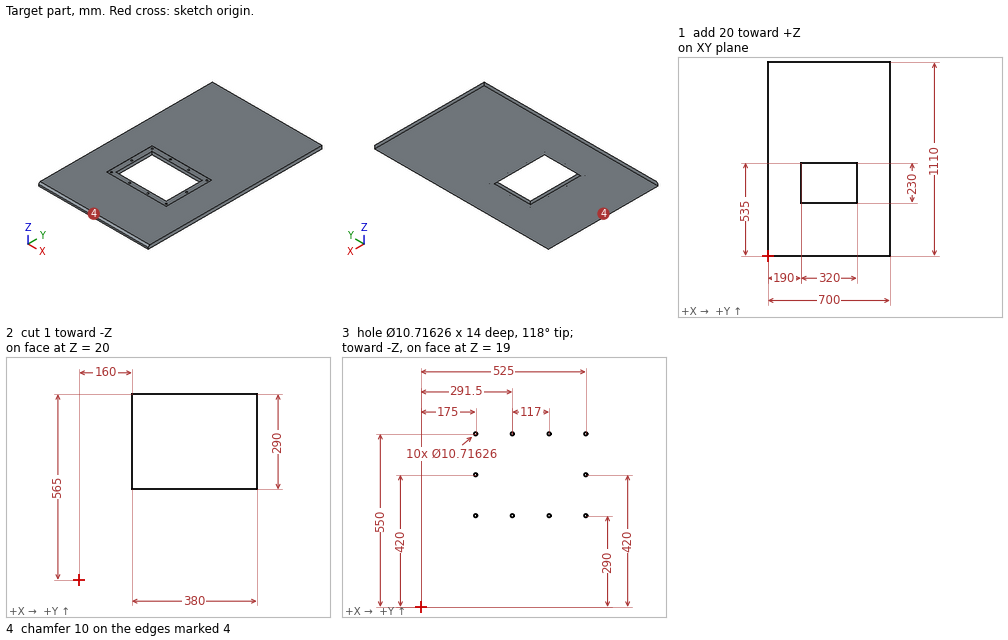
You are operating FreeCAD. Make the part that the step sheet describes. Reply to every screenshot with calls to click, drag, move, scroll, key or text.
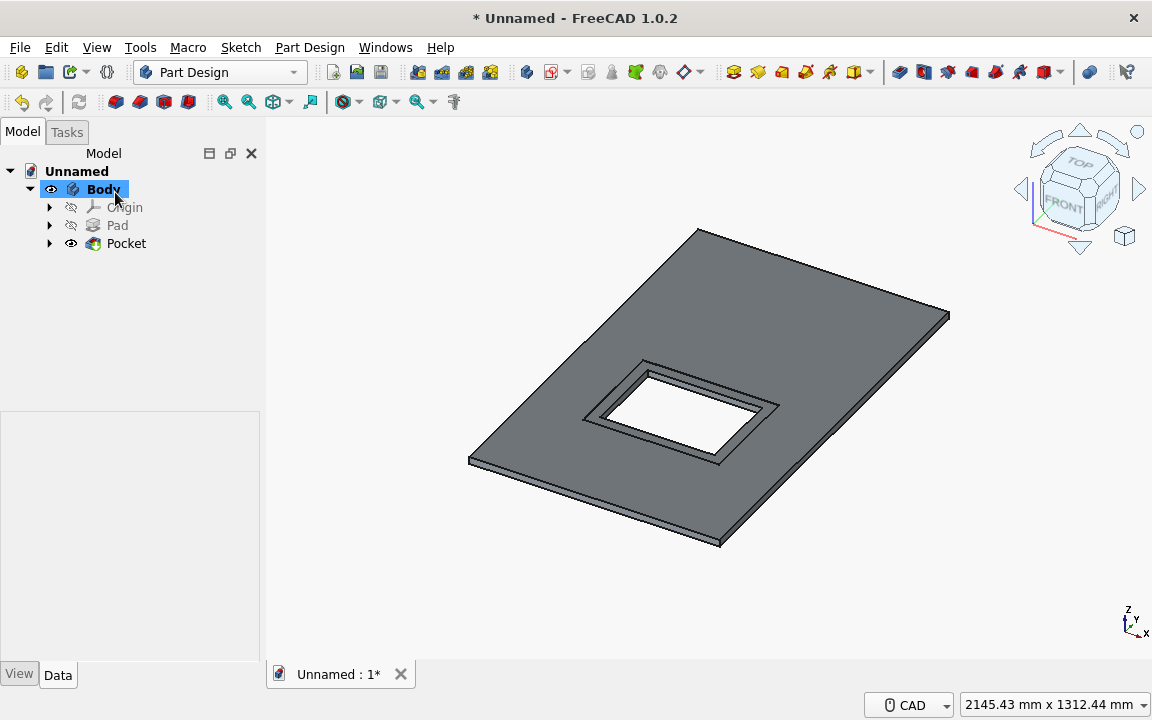
scroll(714, 456, up, 6)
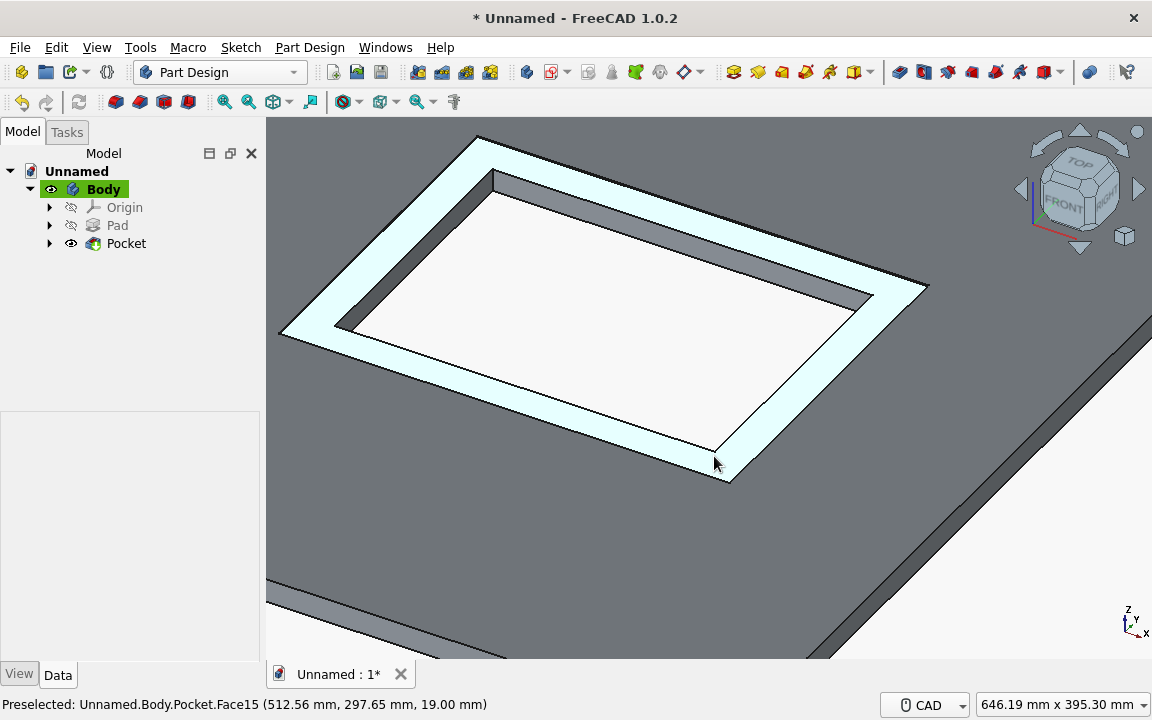
click(712, 458)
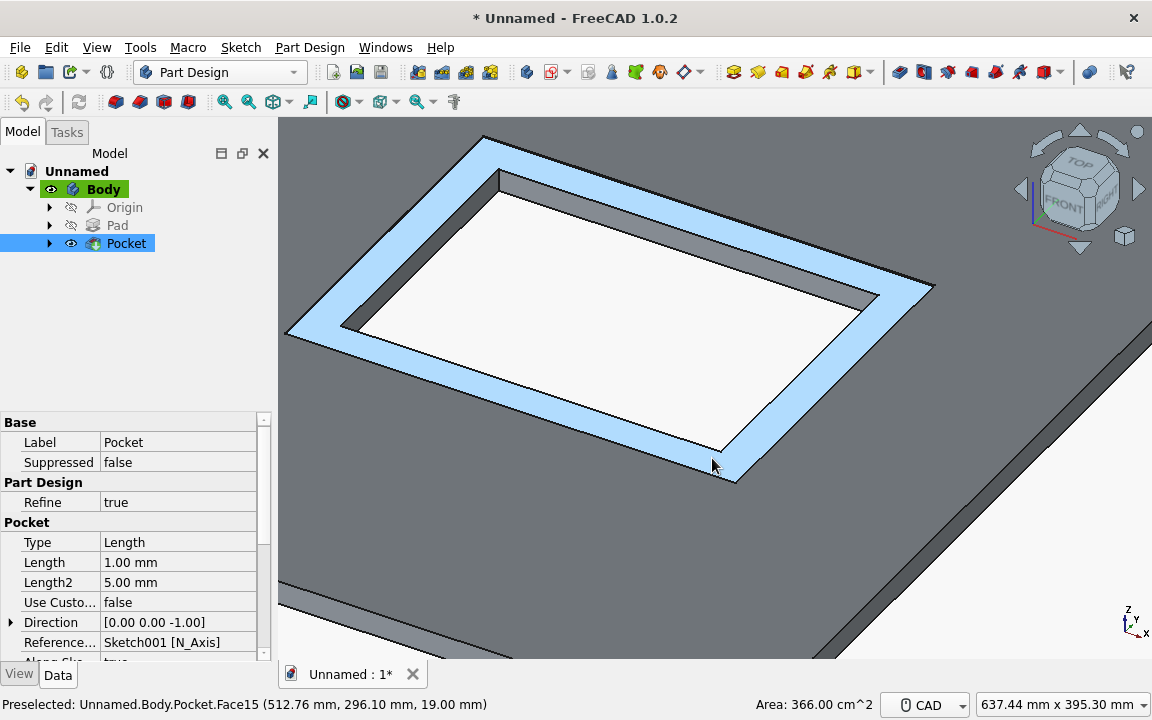
click(552, 72)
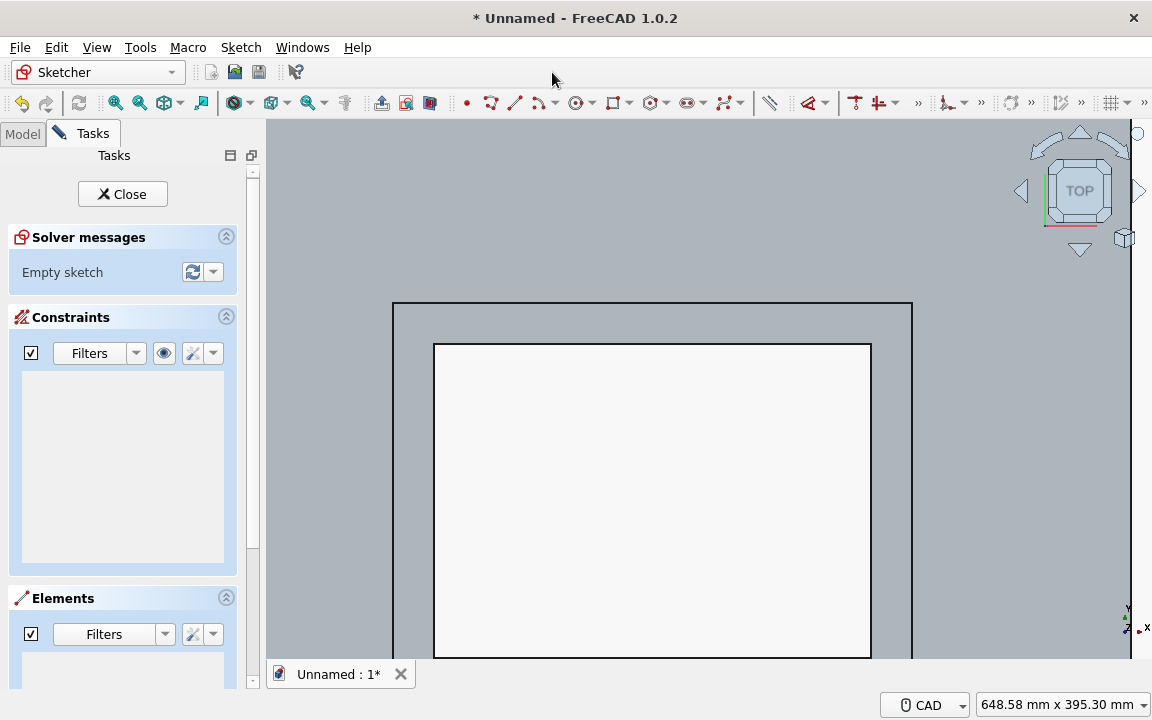
scroll(725, 147, down, 4)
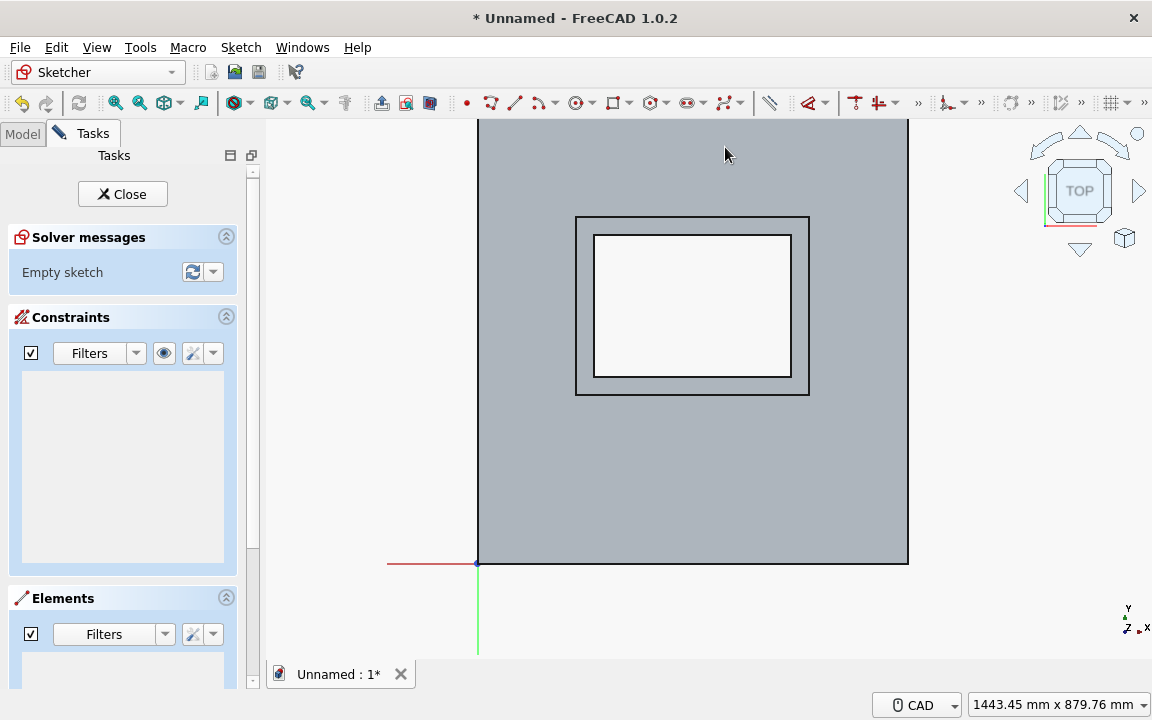
click(576, 104)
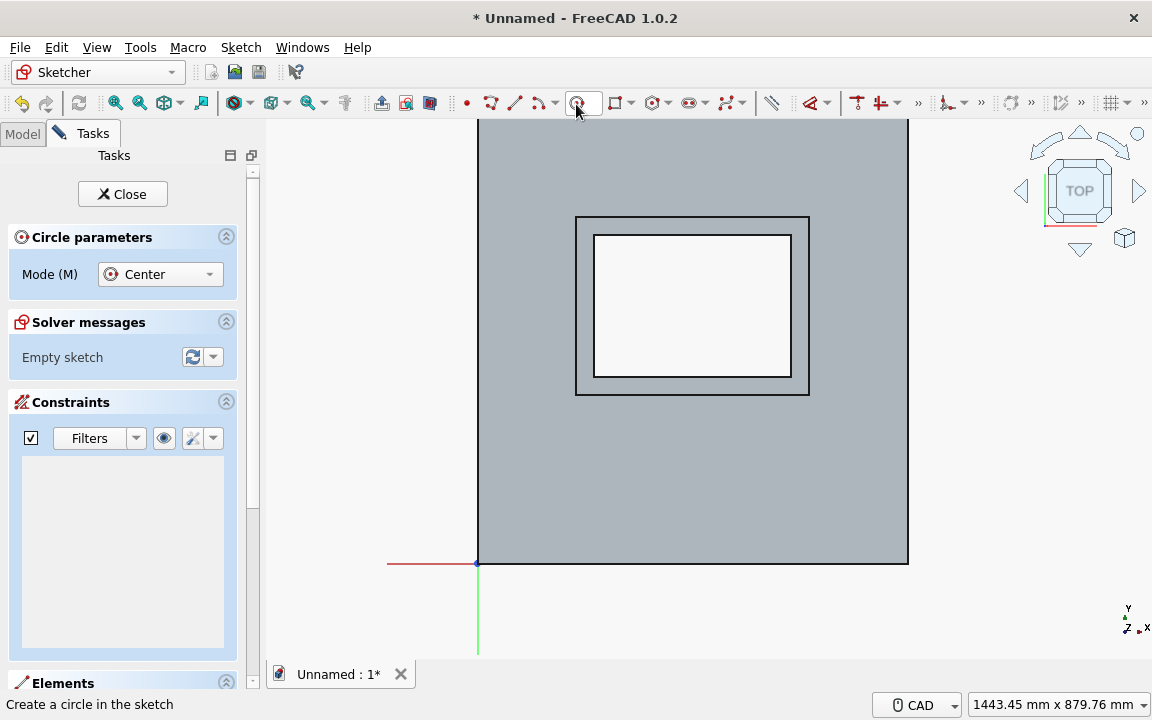
scroll(585, 226, up, 10)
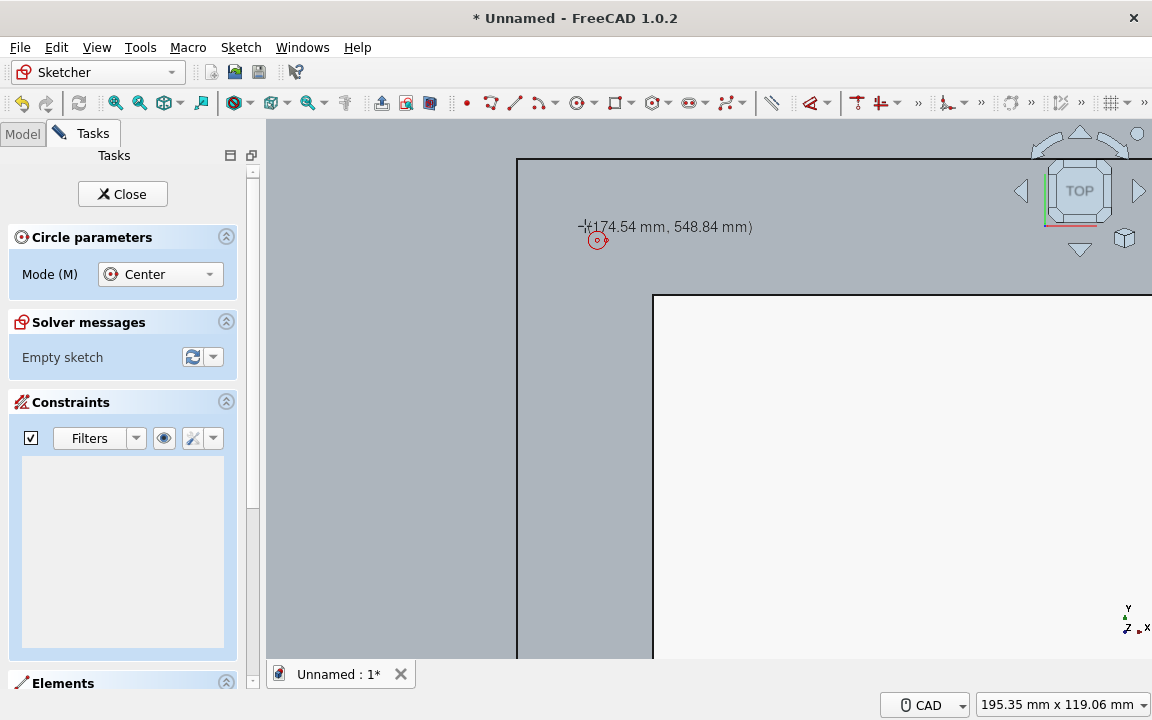
scroll(585, 221, down, 10)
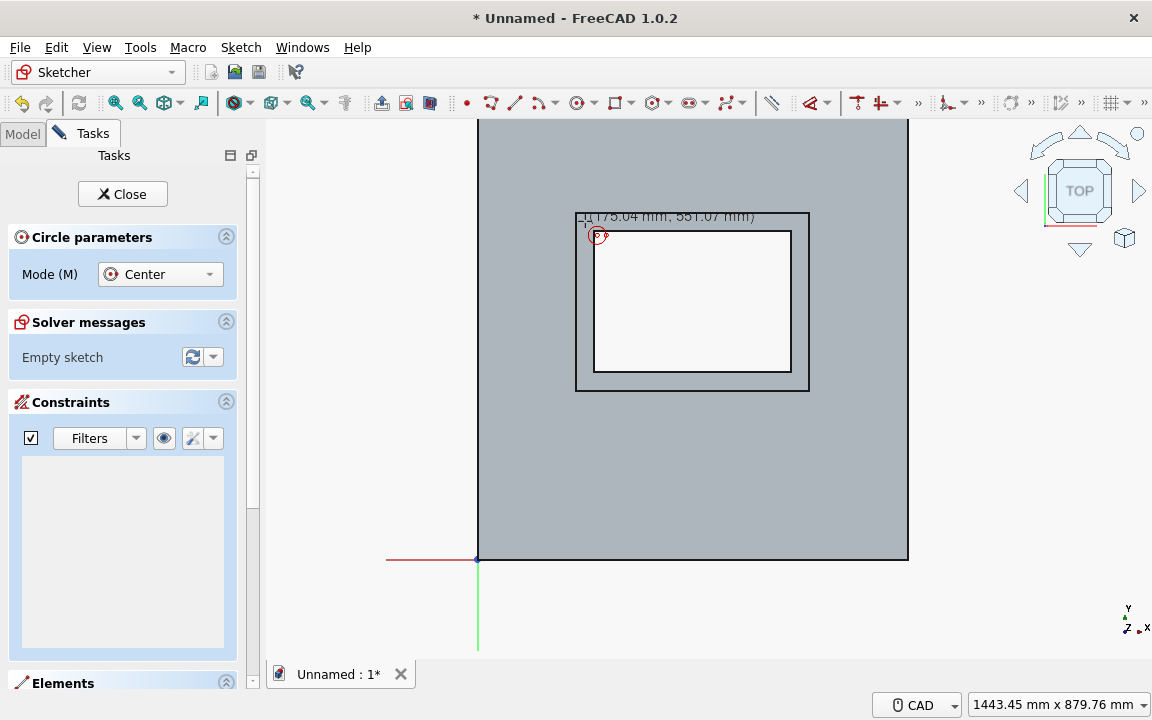
click(585, 222)
move(588, 220)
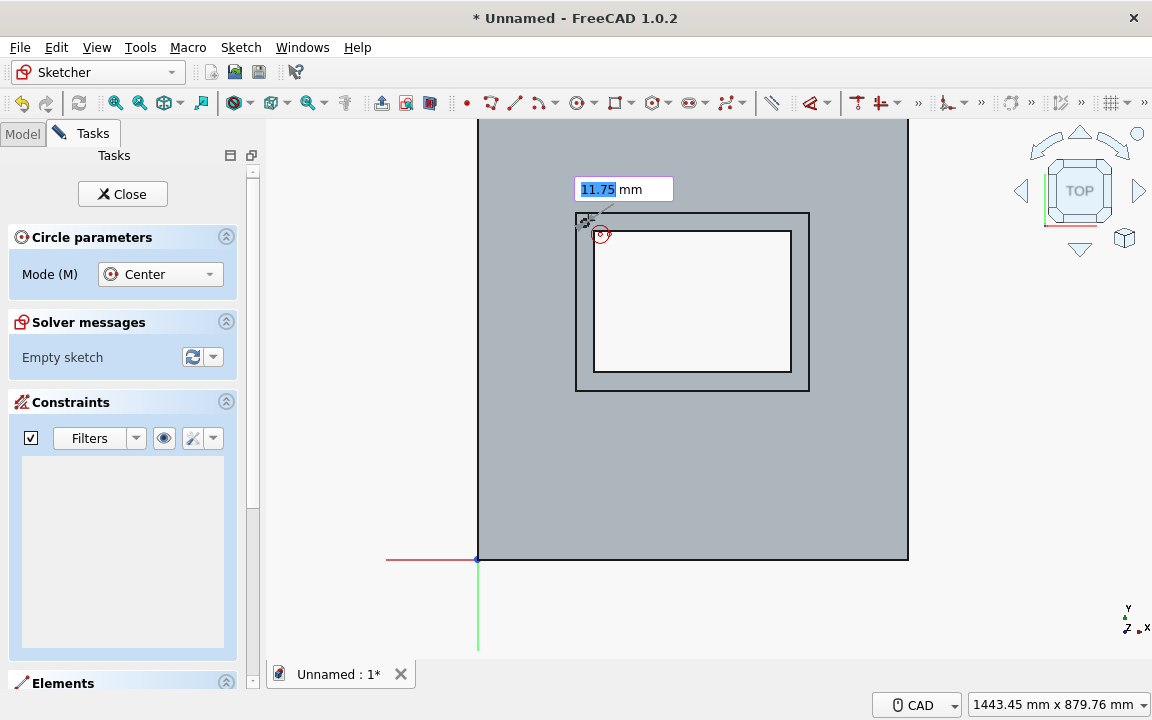
text(10.71626)
key(Return)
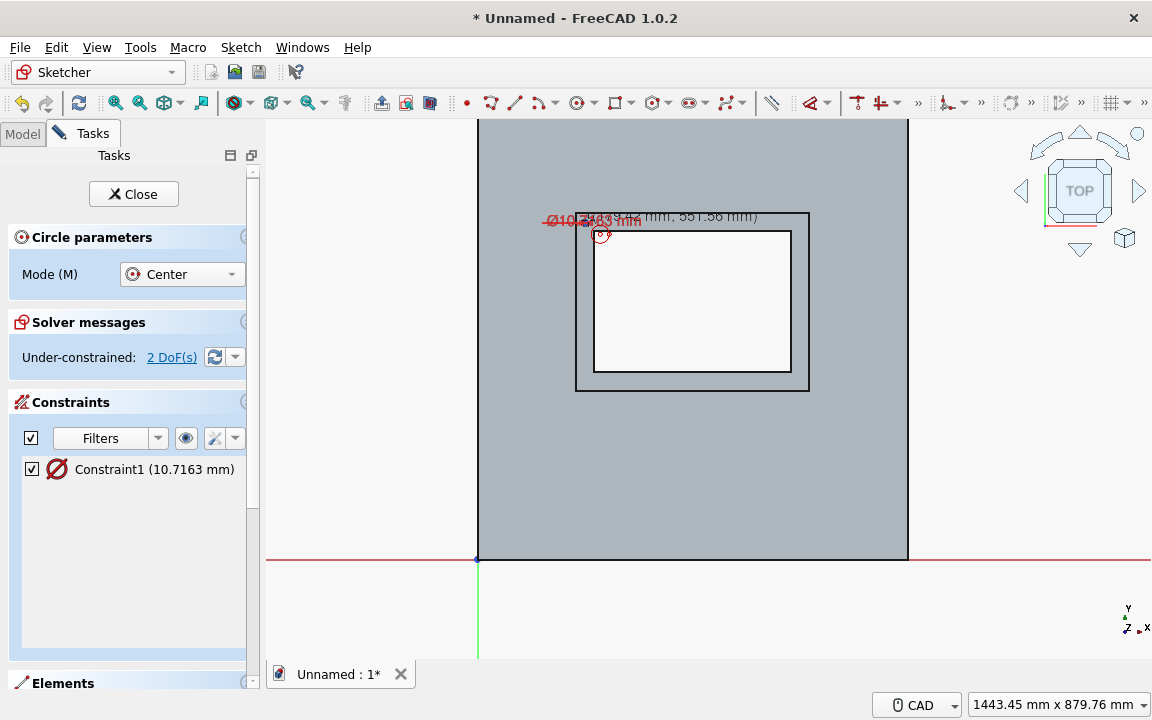
scroll(657, 222, up, 10)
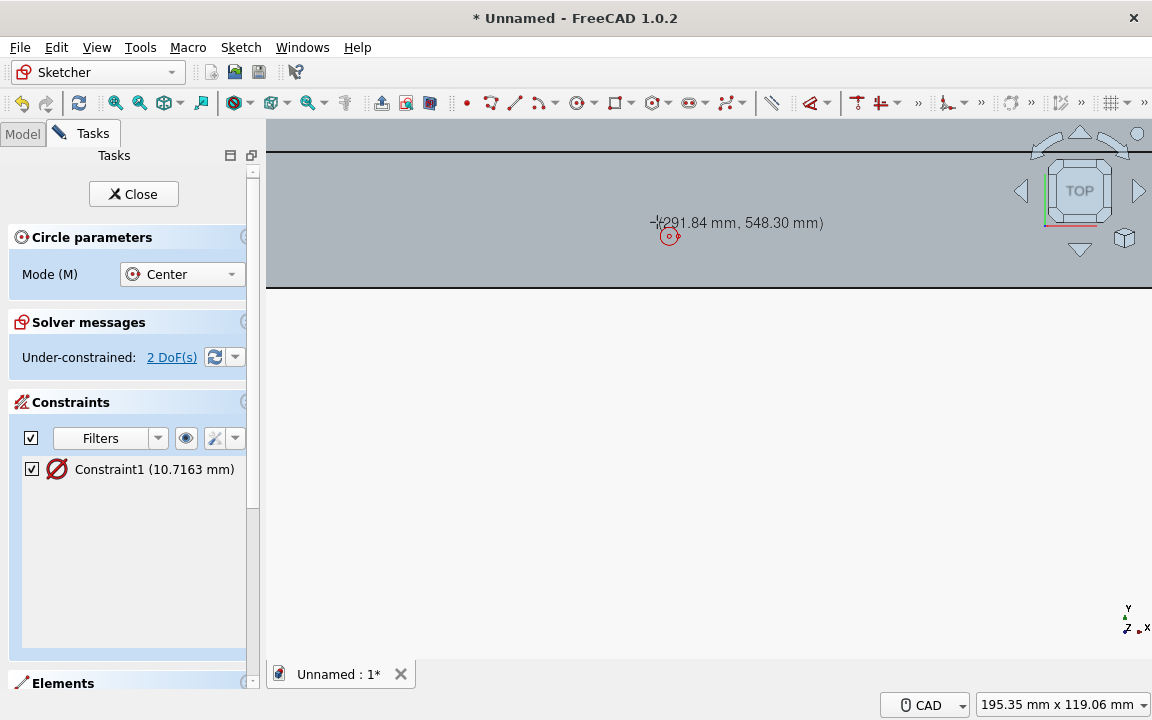
scroll(657, 222, down, 10)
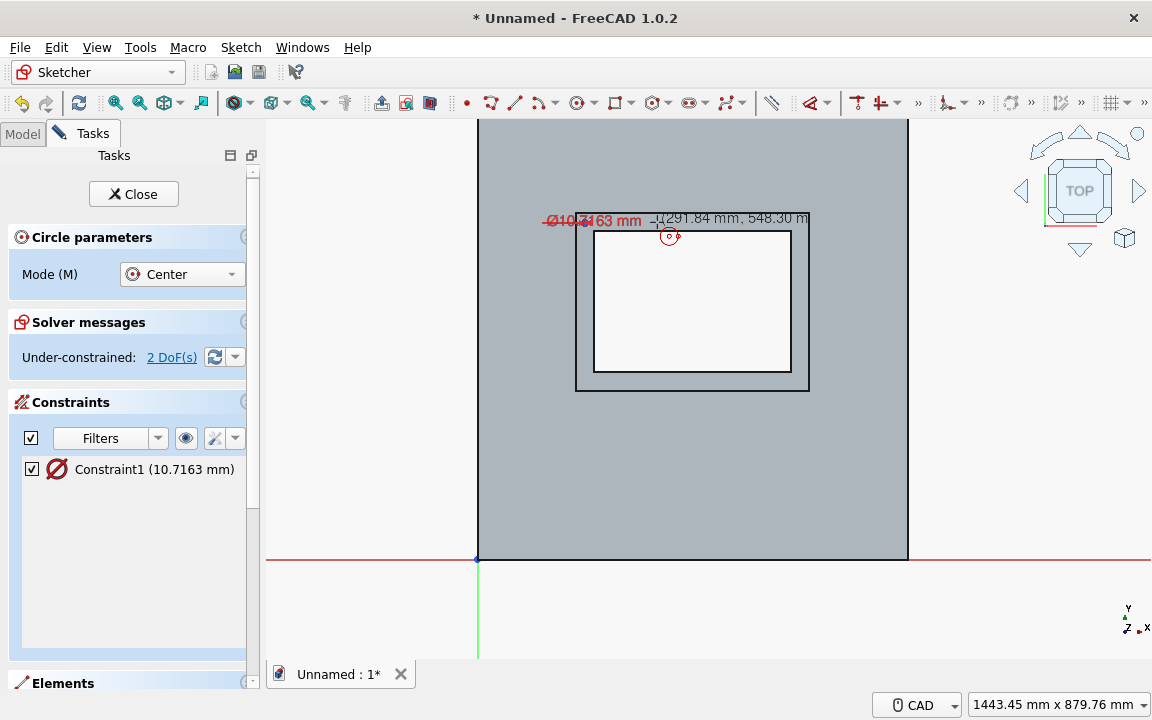
click(657, 222)
move(659, 220)